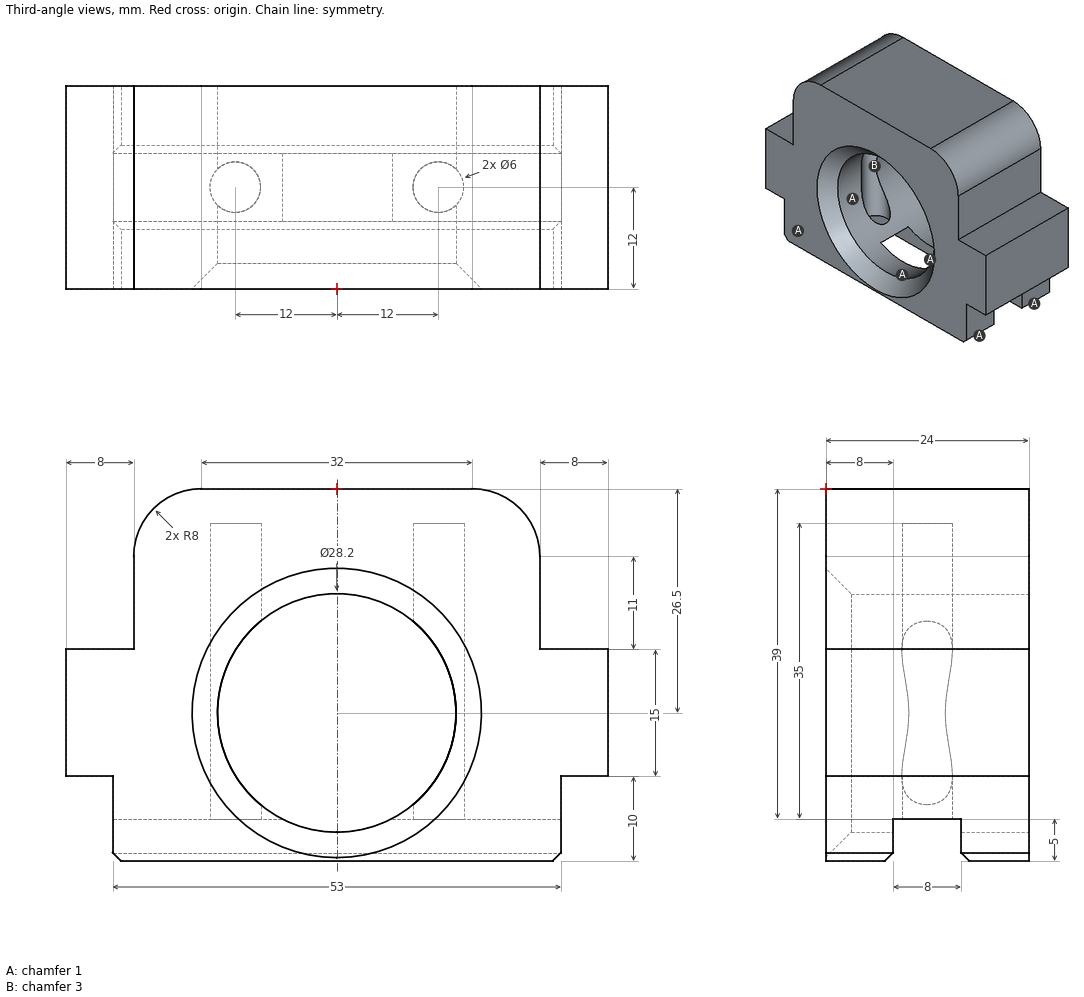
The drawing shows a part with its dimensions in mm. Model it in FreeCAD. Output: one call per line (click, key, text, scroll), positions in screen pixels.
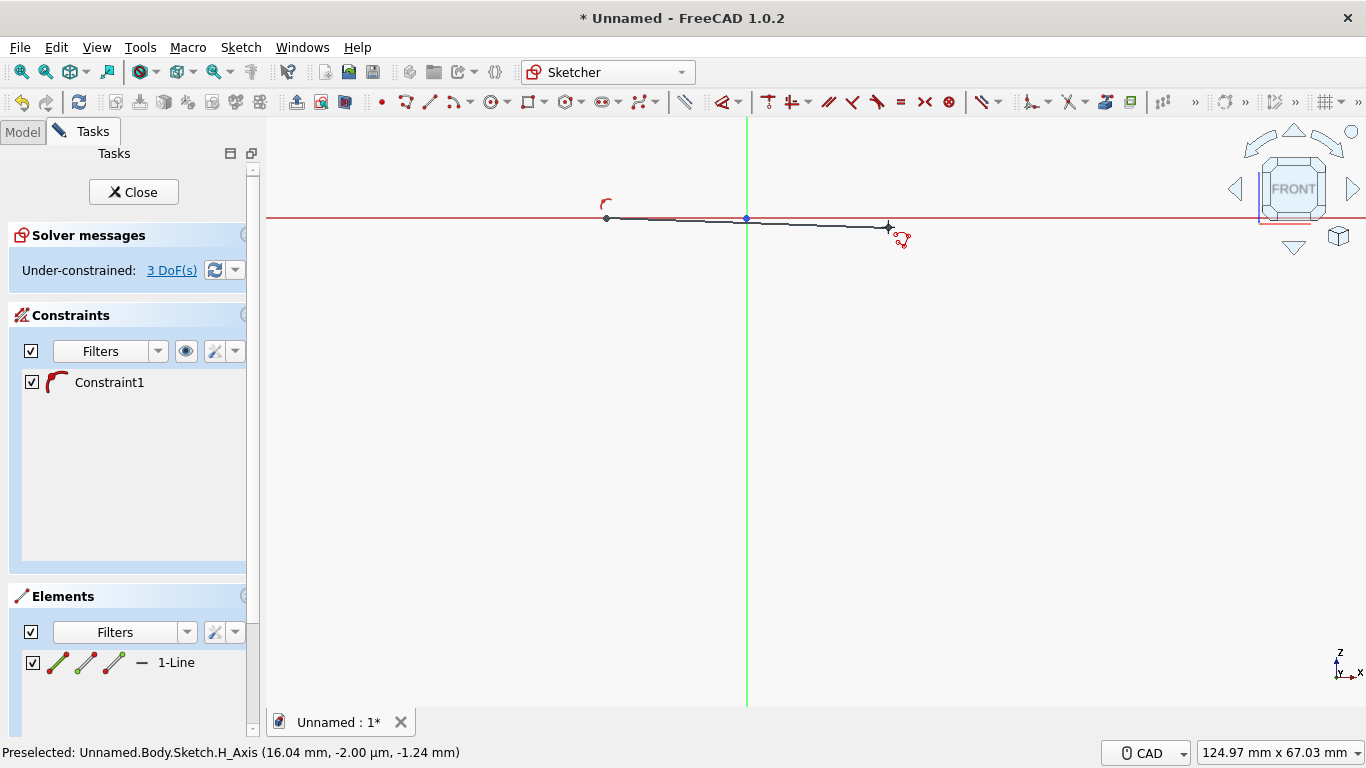
click(958, 288)
click(958, 385)
click(1028, 385)
click(1028, 517)
click(980, 517)
click(980, 605)
click(513, 605)
click(513, 517)
click(465, 517)
click(465, 385)
click(536, 385)
click(536, 288)
right_click(536, 288)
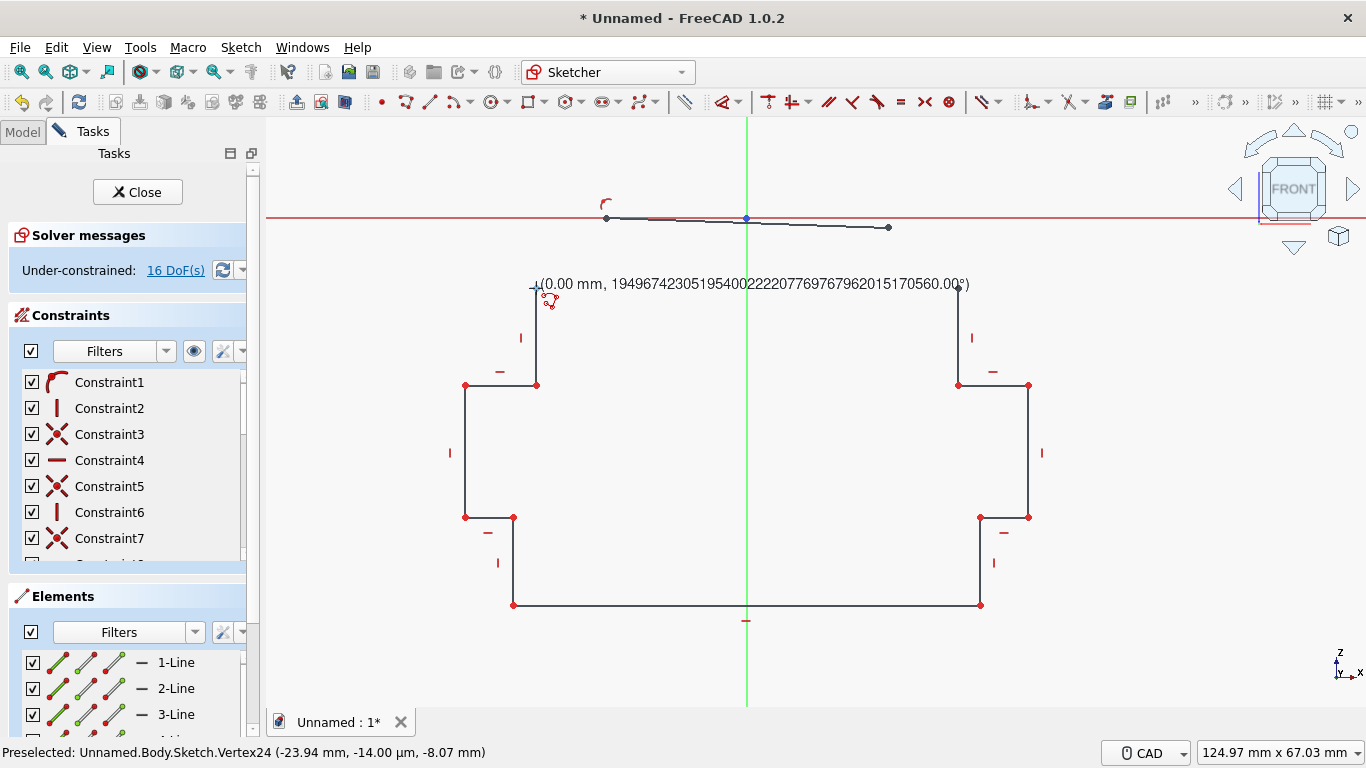
click(472, 102)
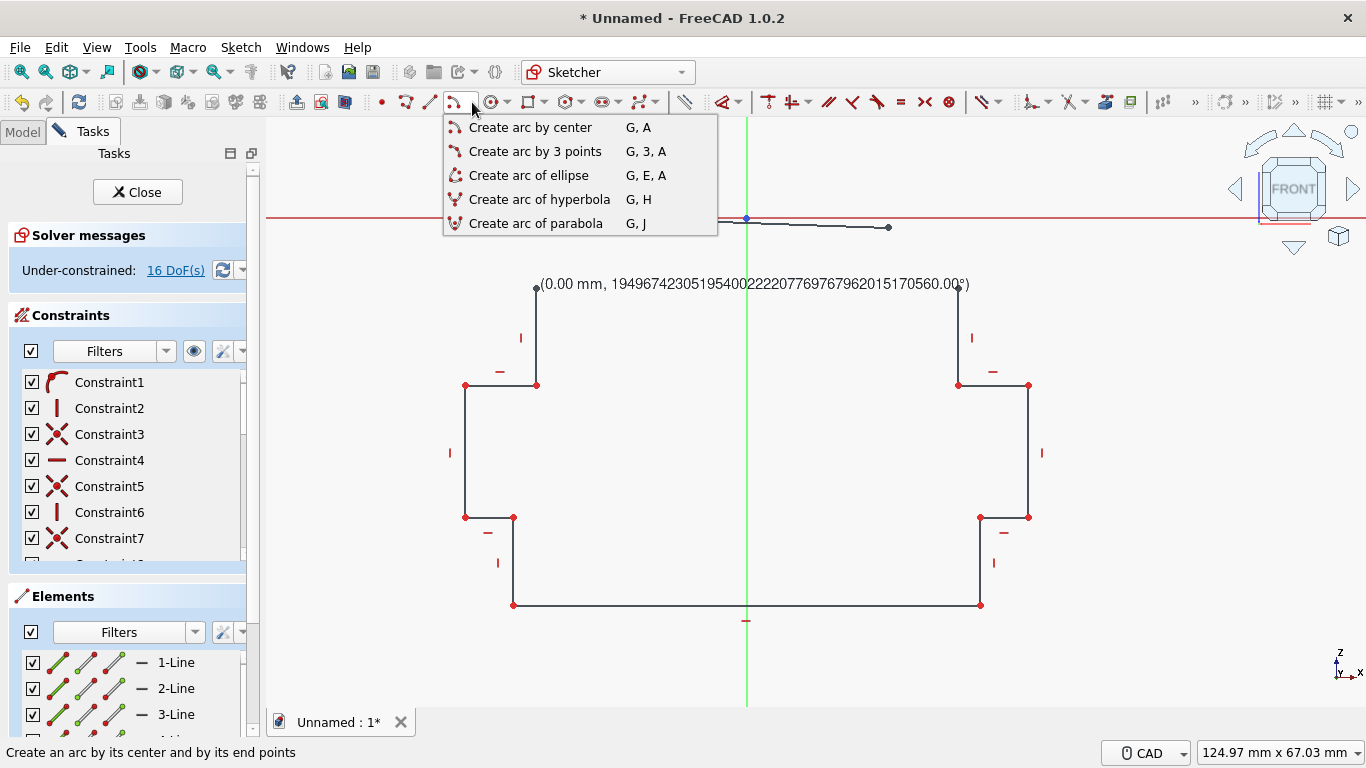
click(580, 151)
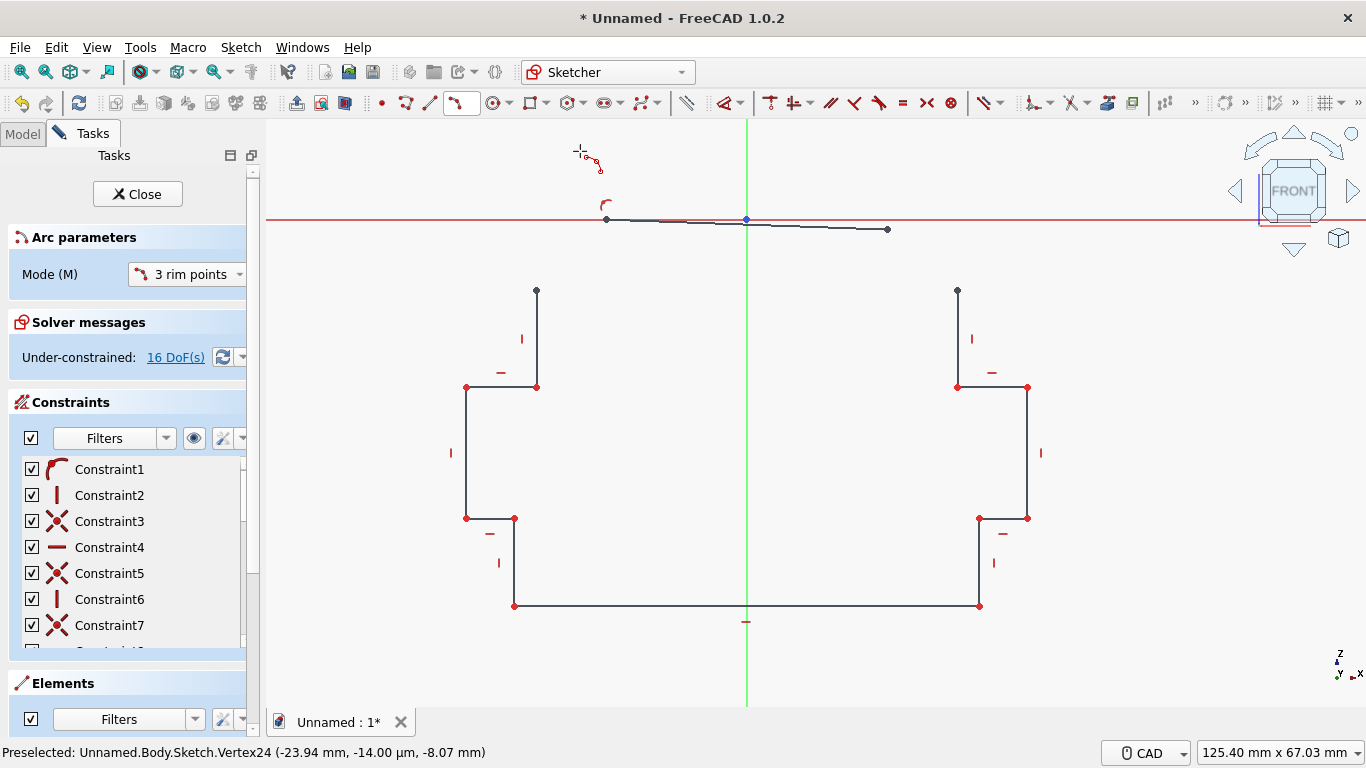
click(888, 230)
click(958, 290)
click(937, 240)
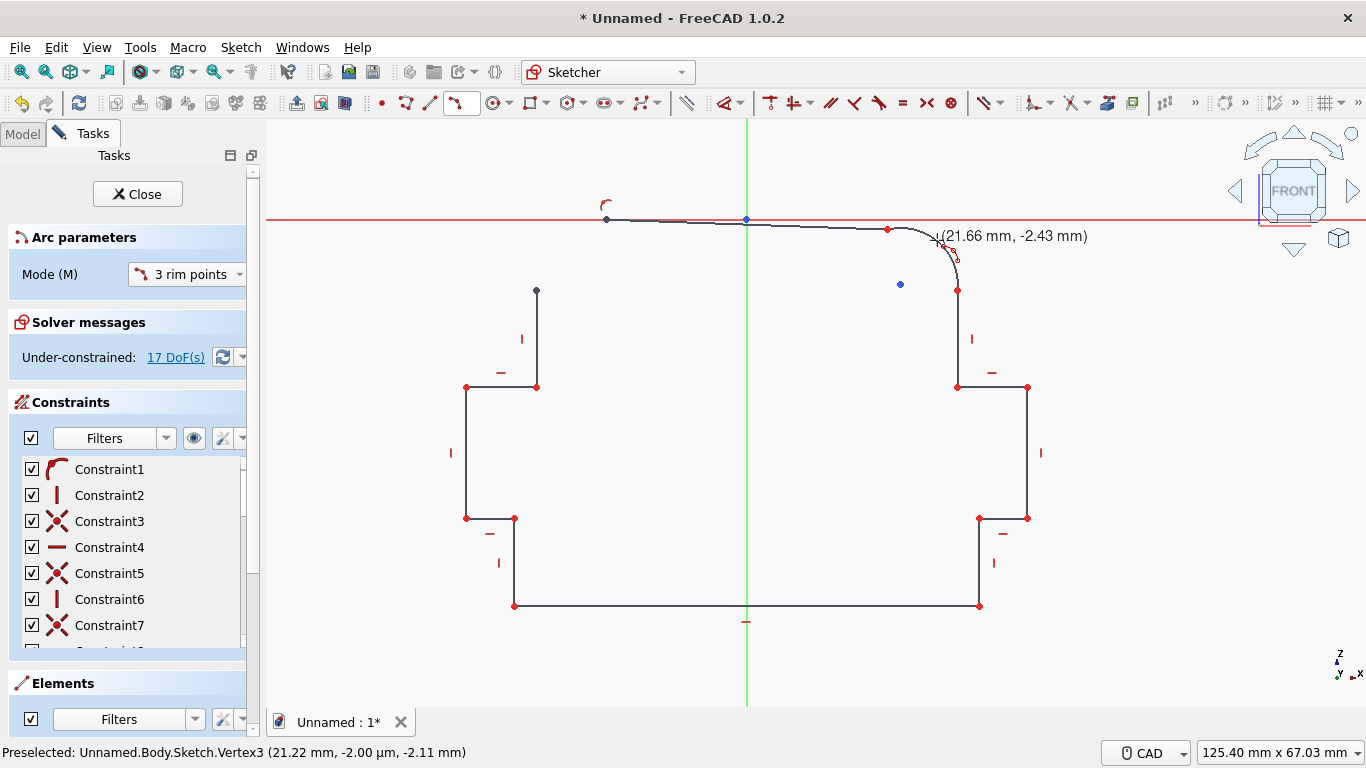
click(537, 290)
click(607, 220)
click(557, 240)
key(Escape)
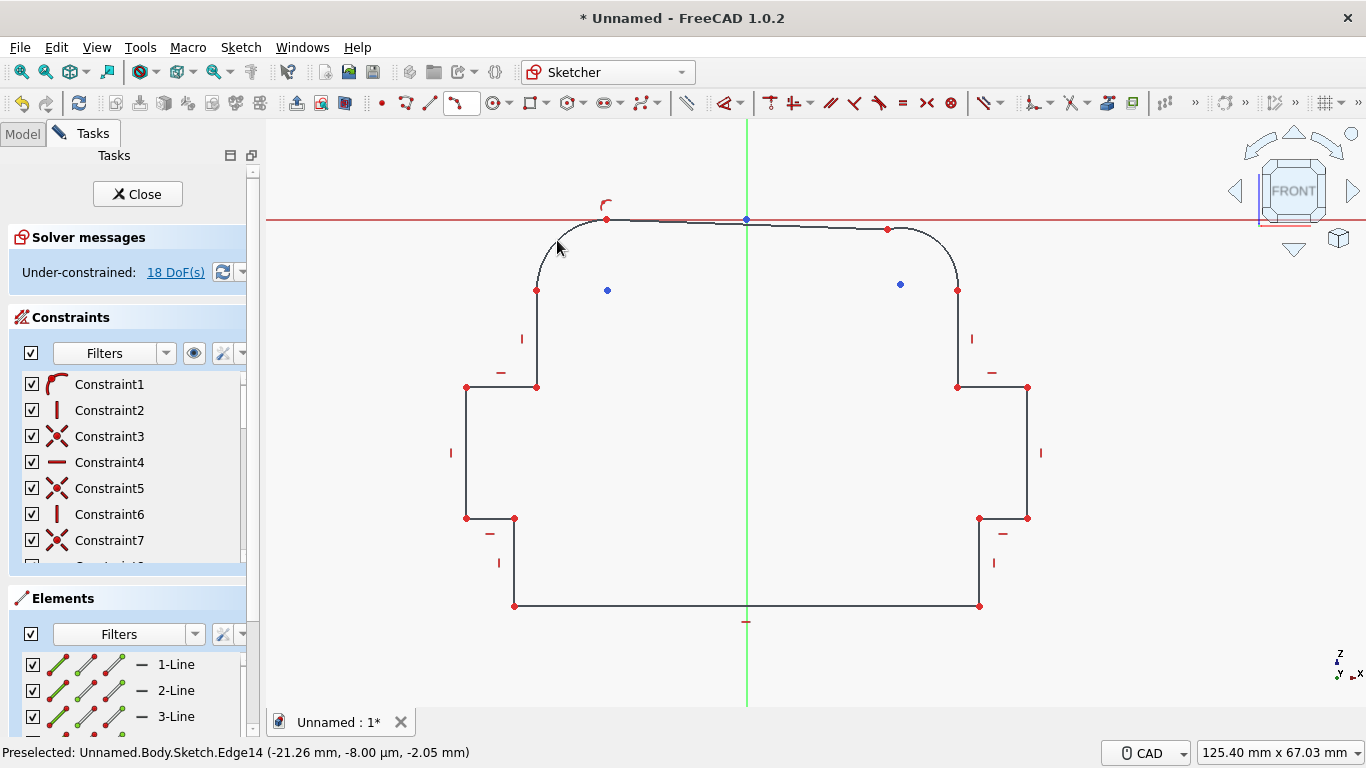
click(691, 223)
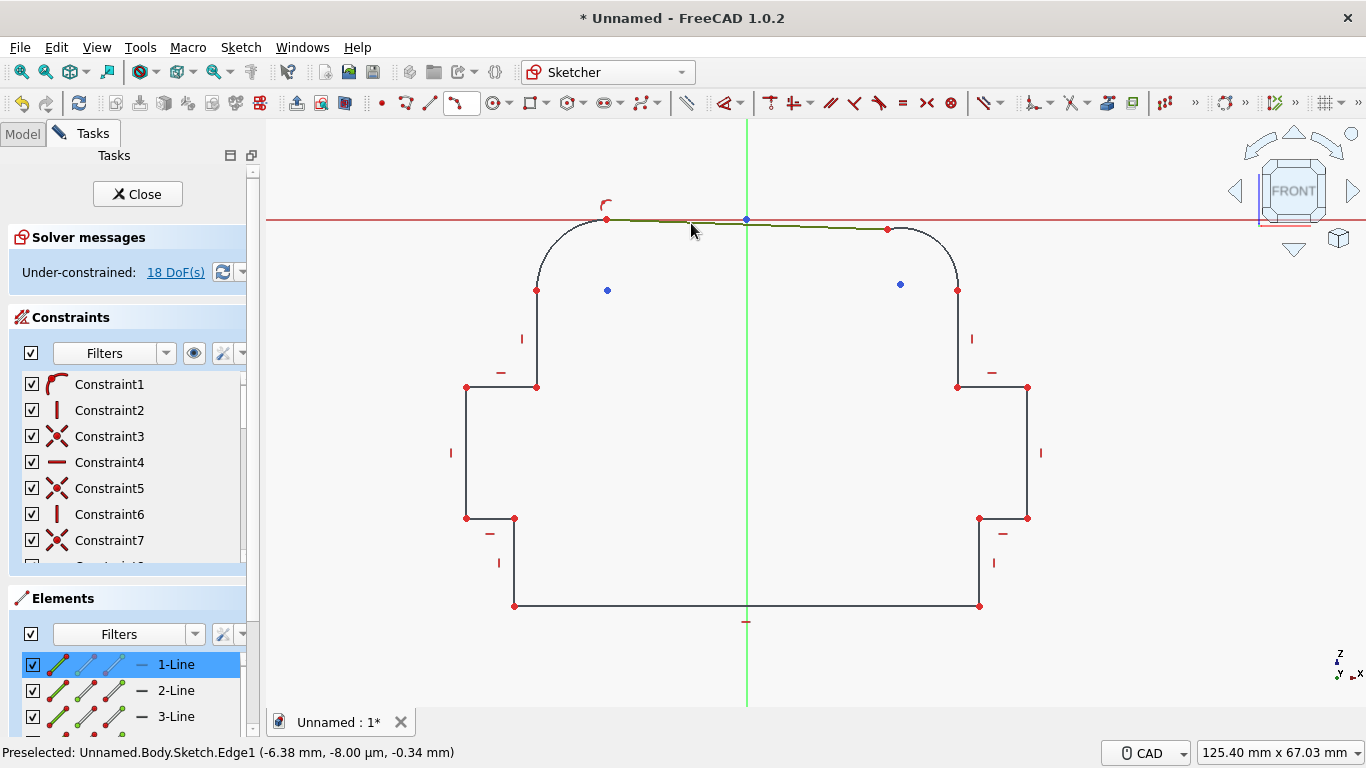
click(952, 259)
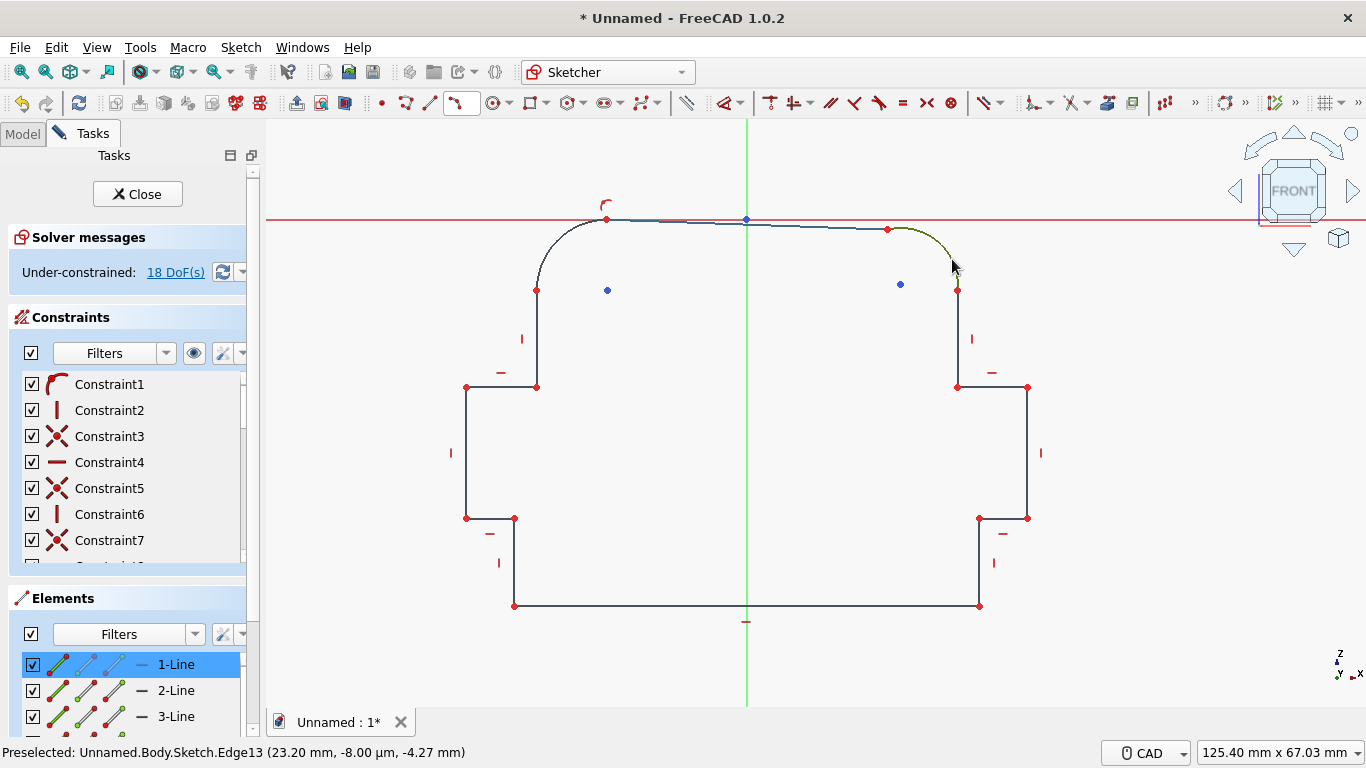
click(880, 104)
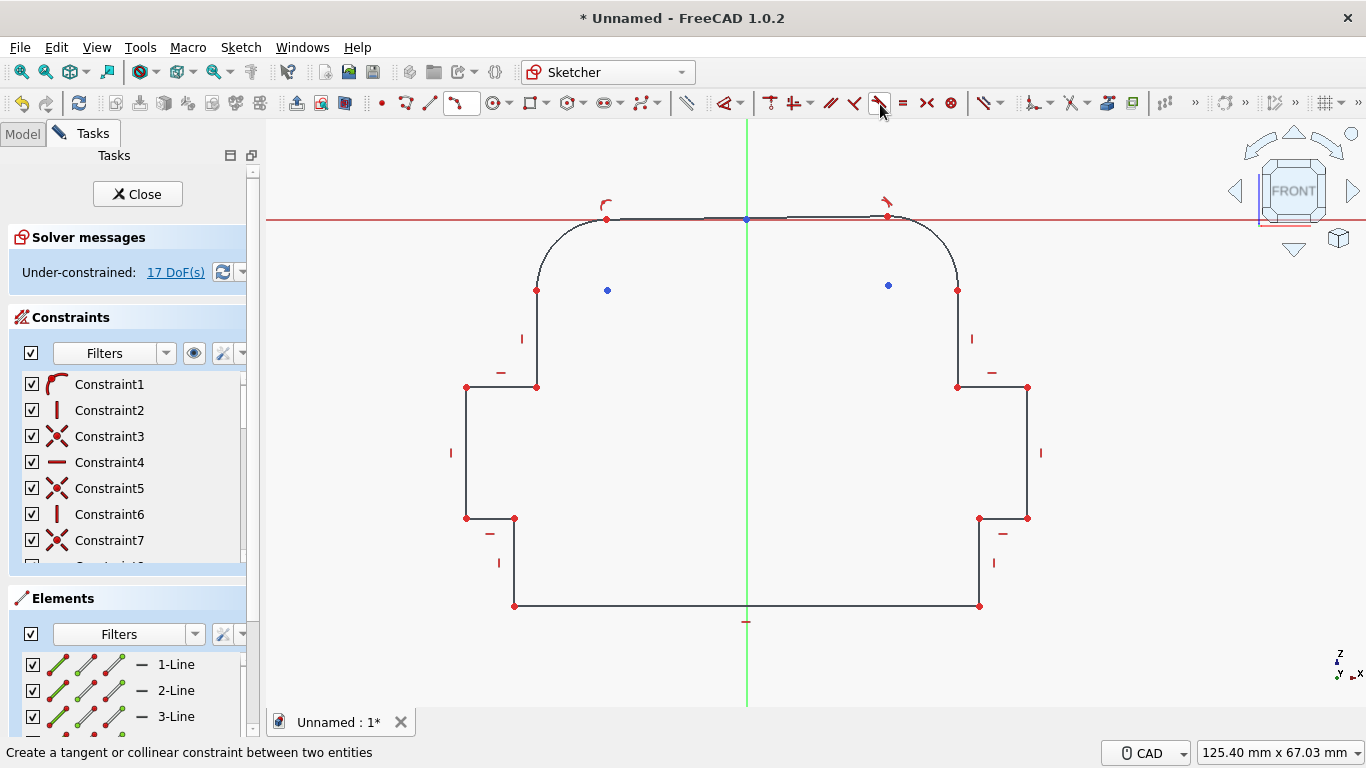
click(691, 219)